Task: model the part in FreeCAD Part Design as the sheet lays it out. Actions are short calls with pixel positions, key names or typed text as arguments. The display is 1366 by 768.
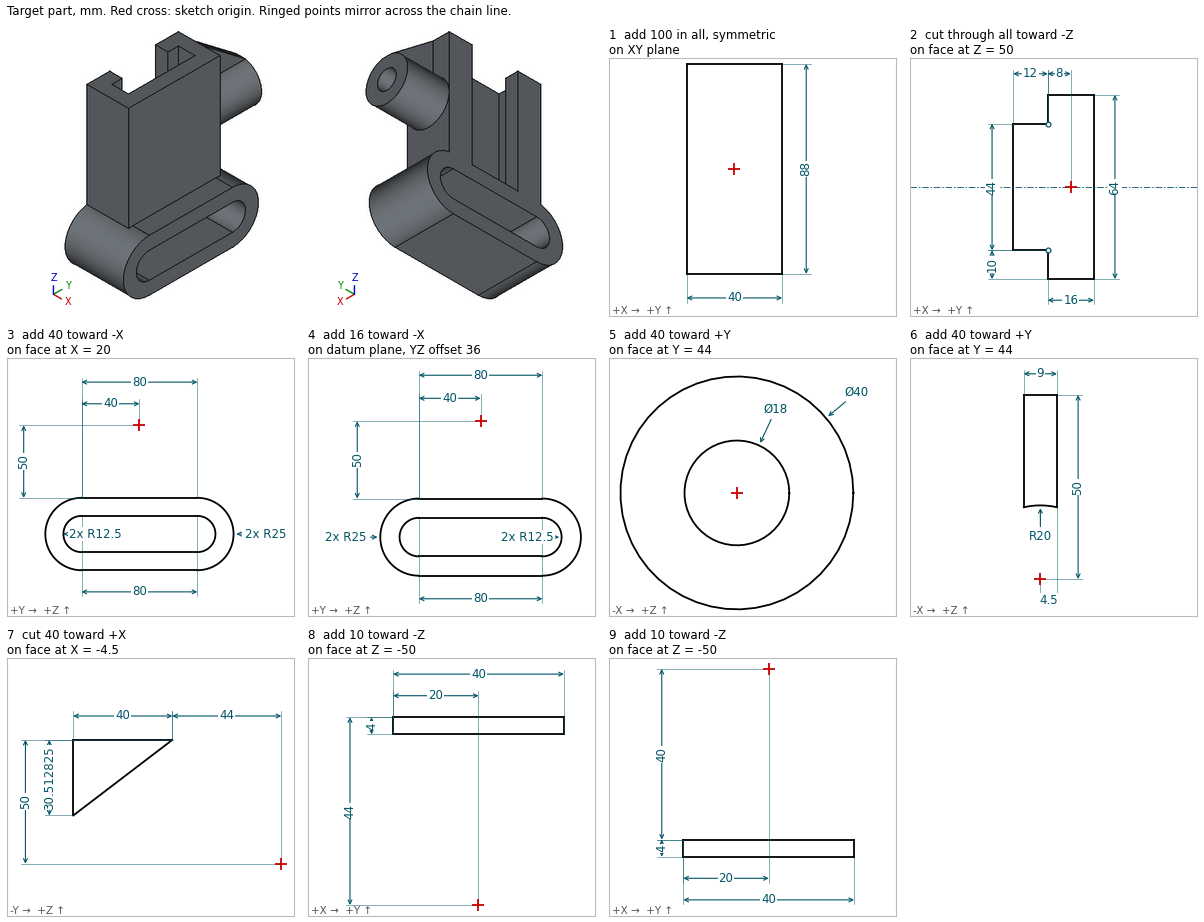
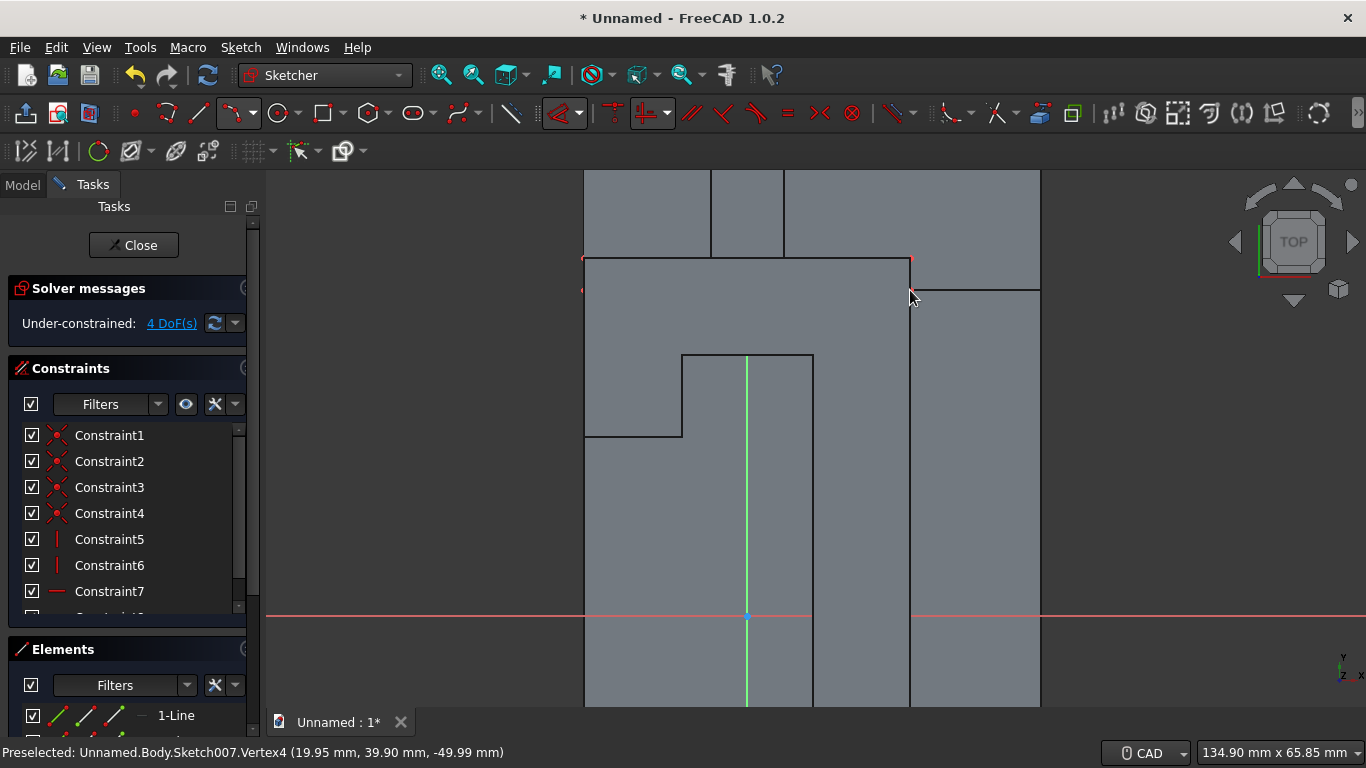
scroll(584, 269, up, 2)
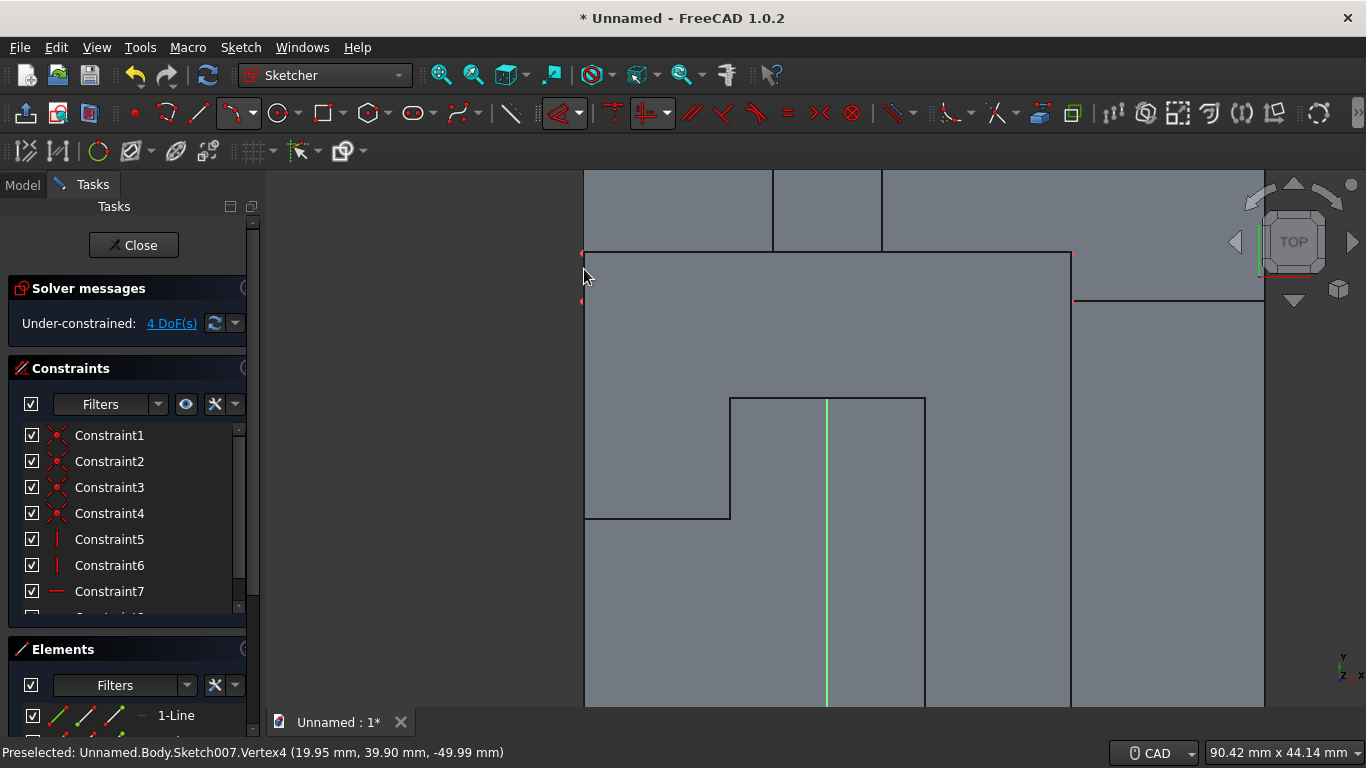
click(584, 268)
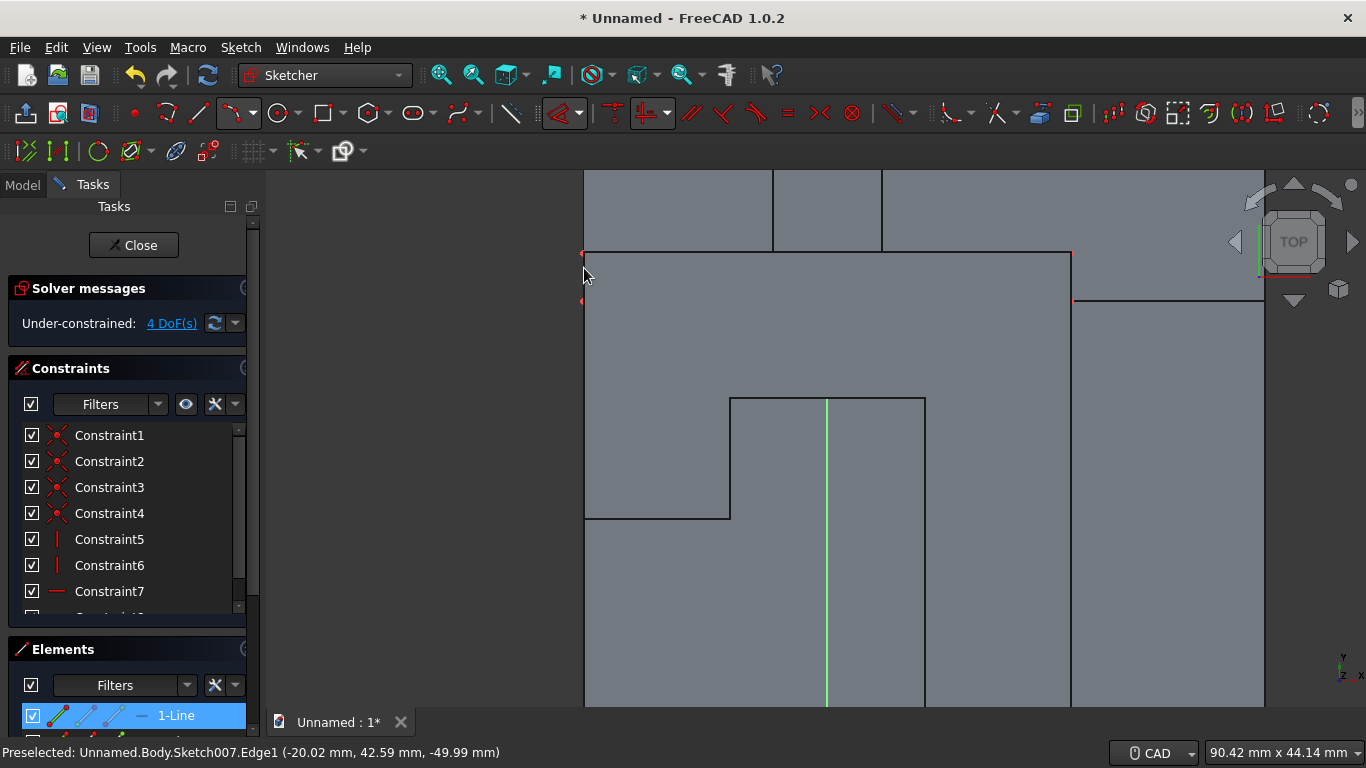
key(i)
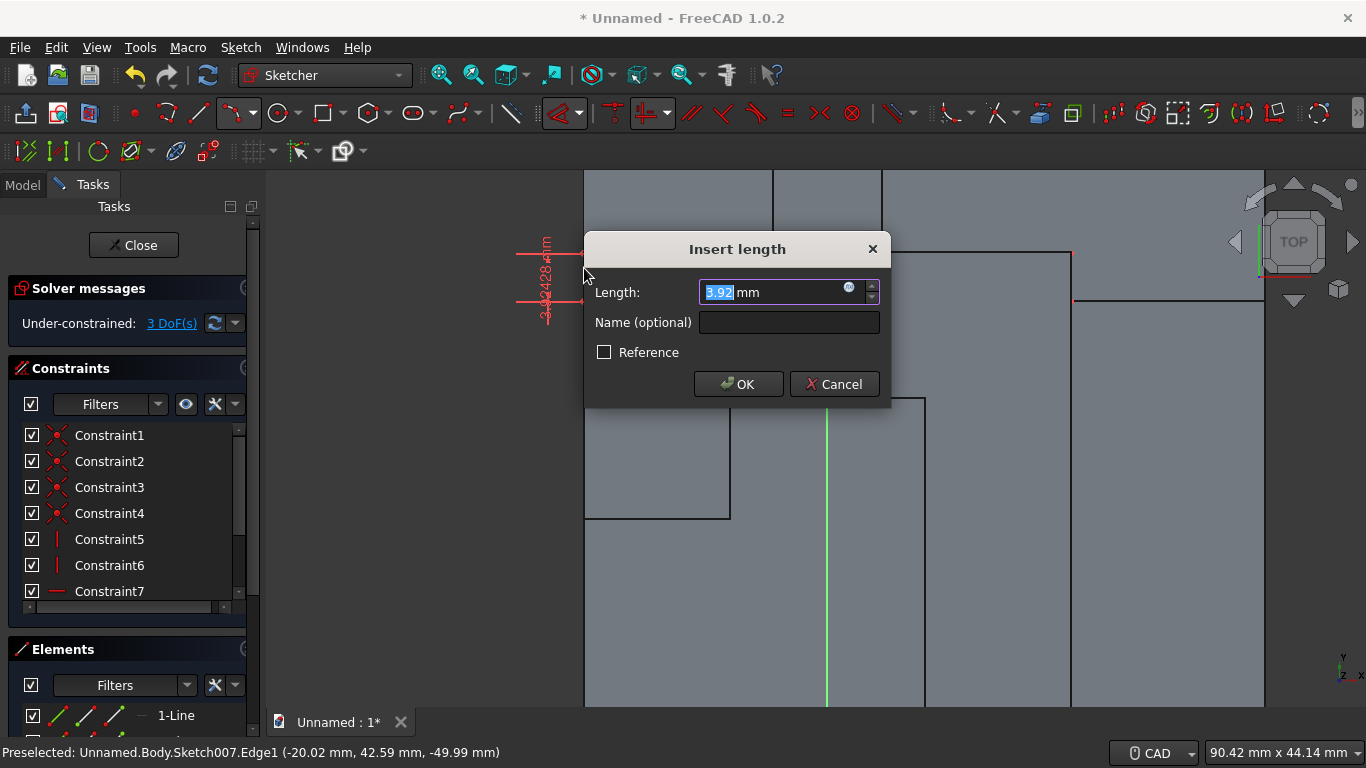
text(4)
key(Return)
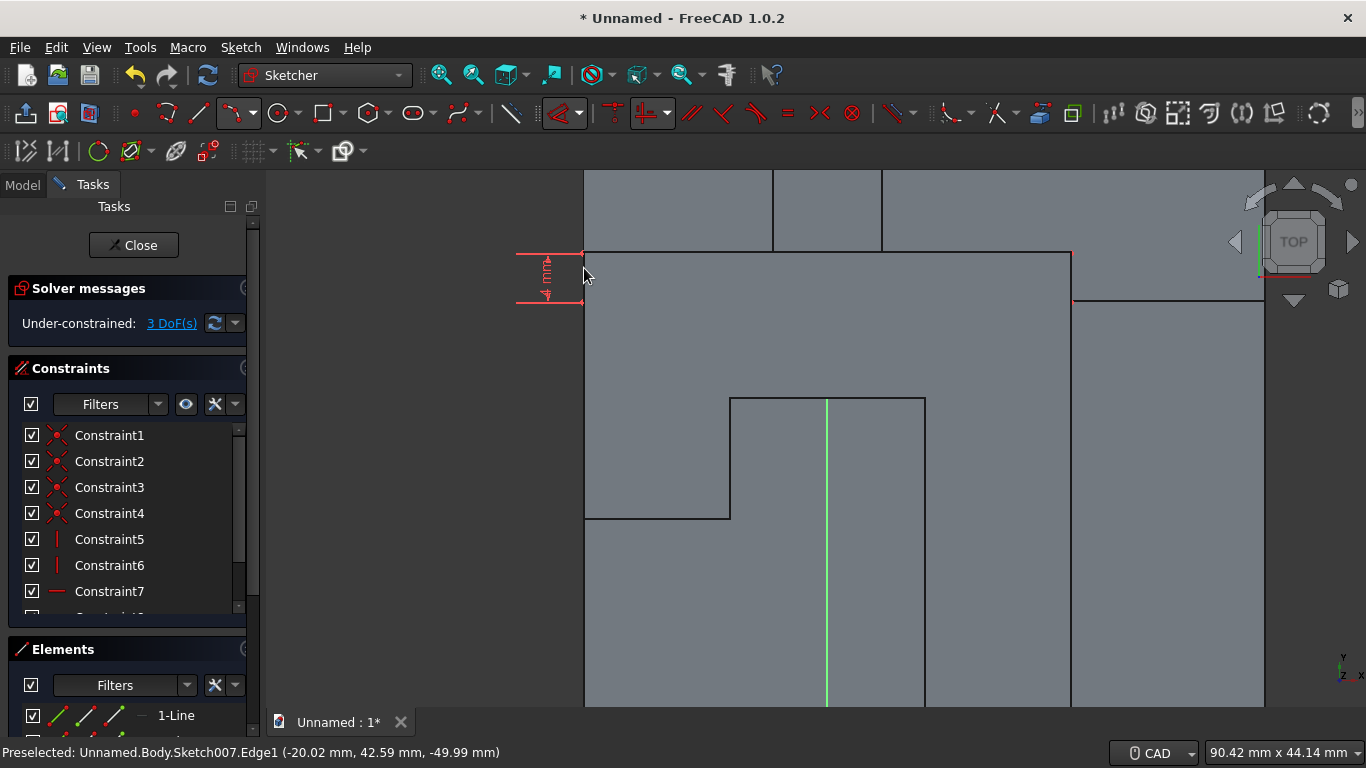
click(730, 303)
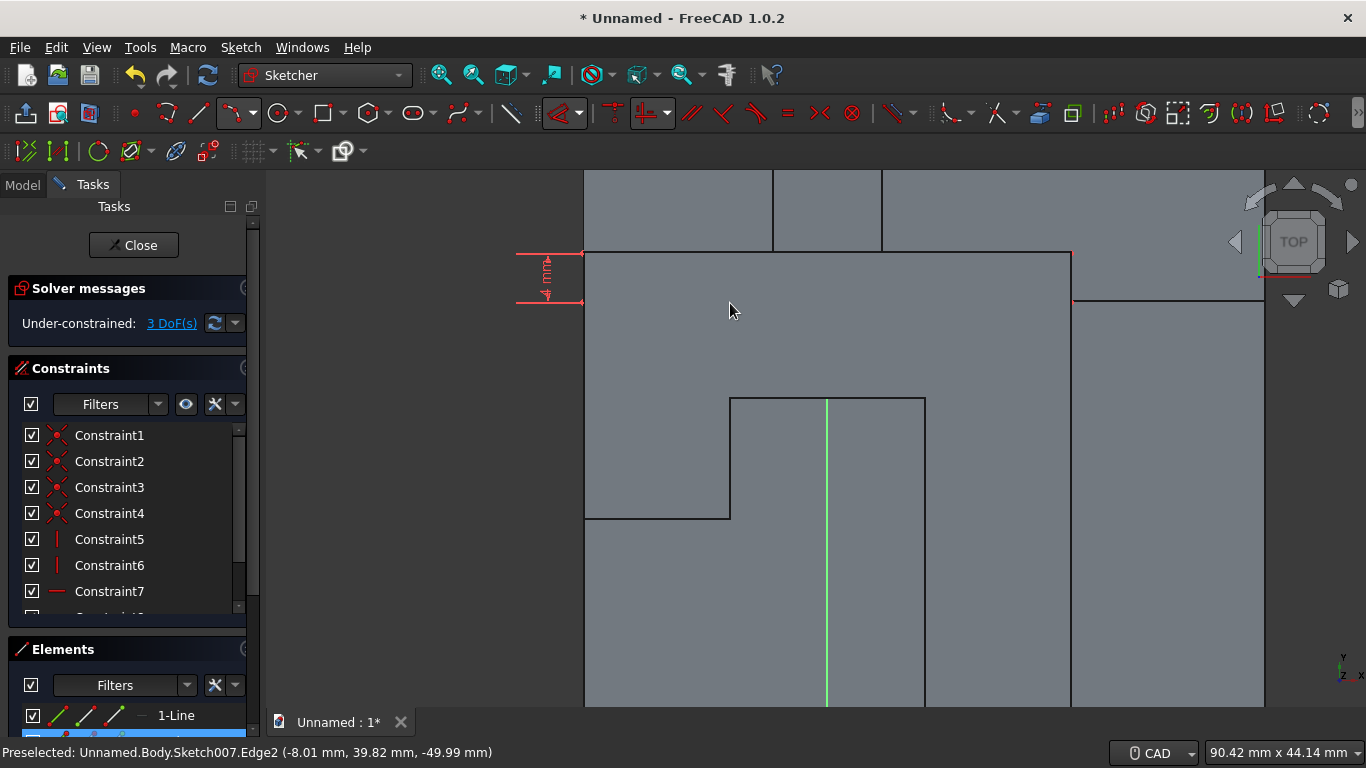
key(l)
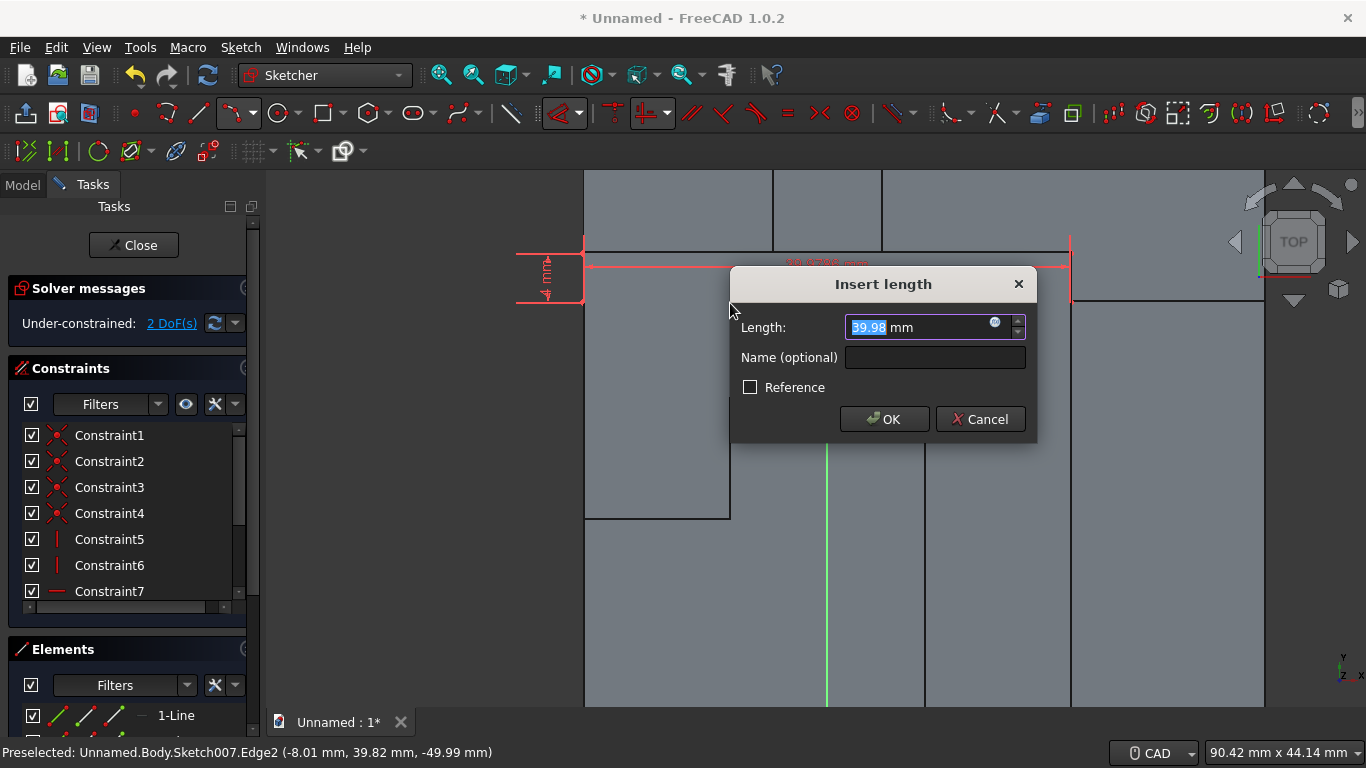
text(40)
key(Return)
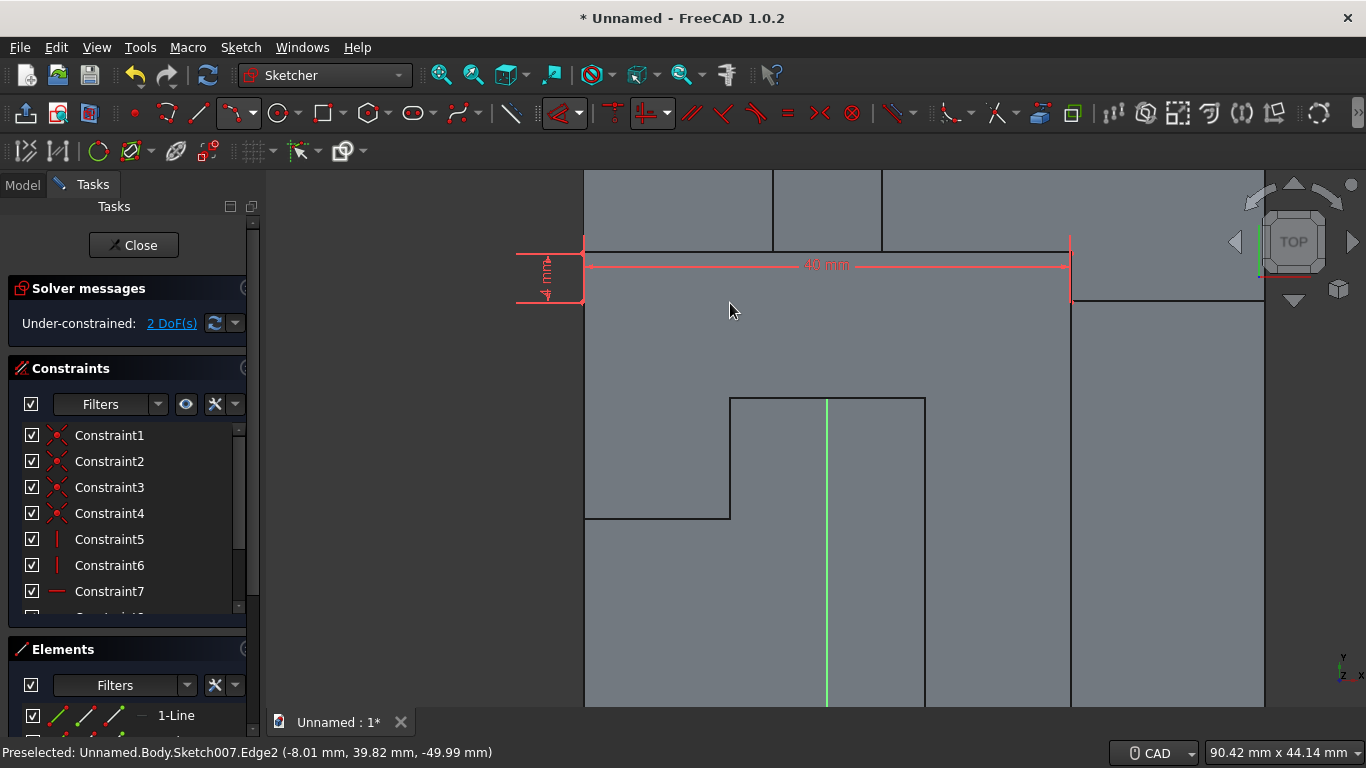
click(584, 254)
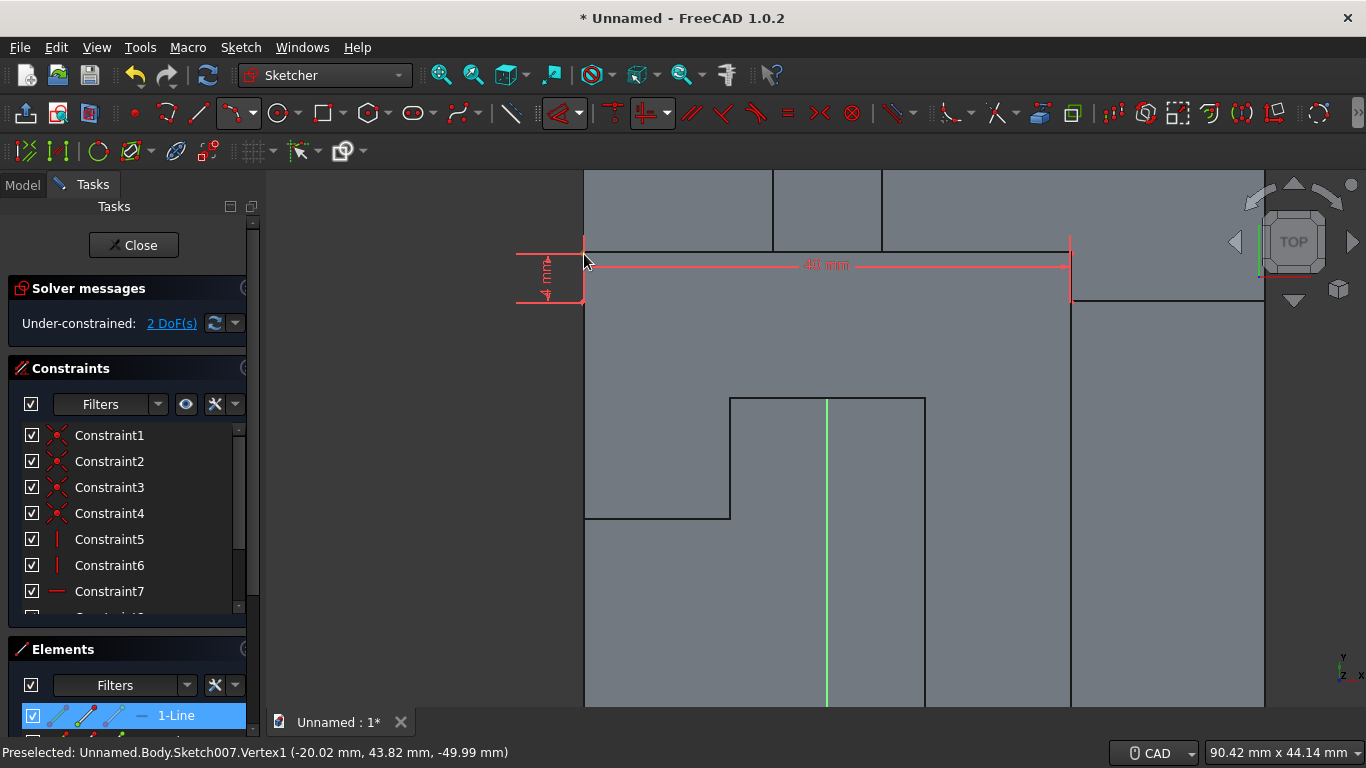
key(l)